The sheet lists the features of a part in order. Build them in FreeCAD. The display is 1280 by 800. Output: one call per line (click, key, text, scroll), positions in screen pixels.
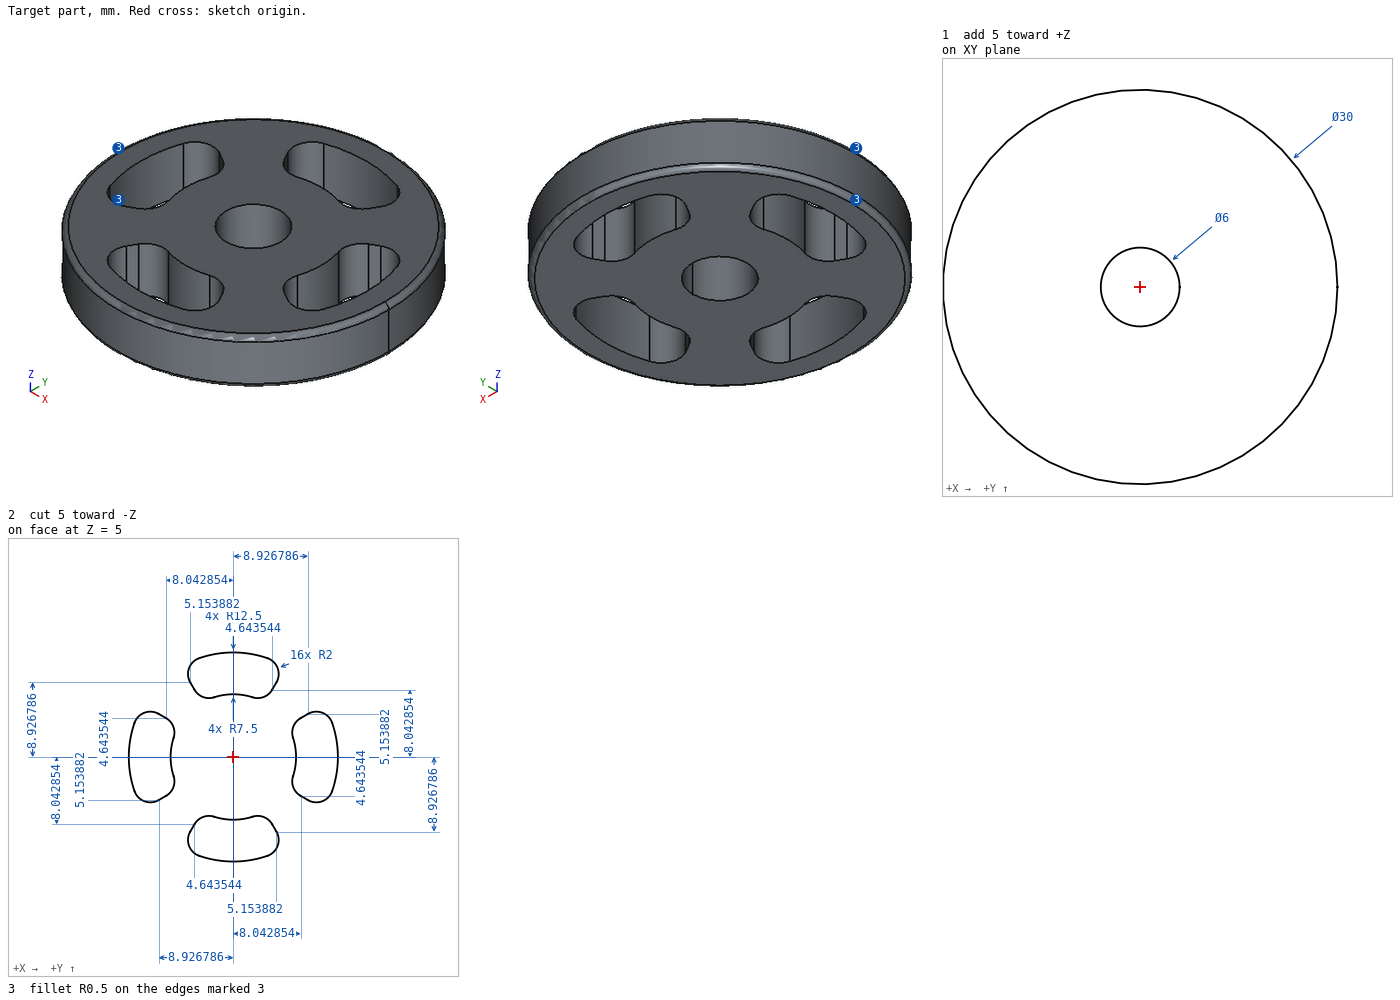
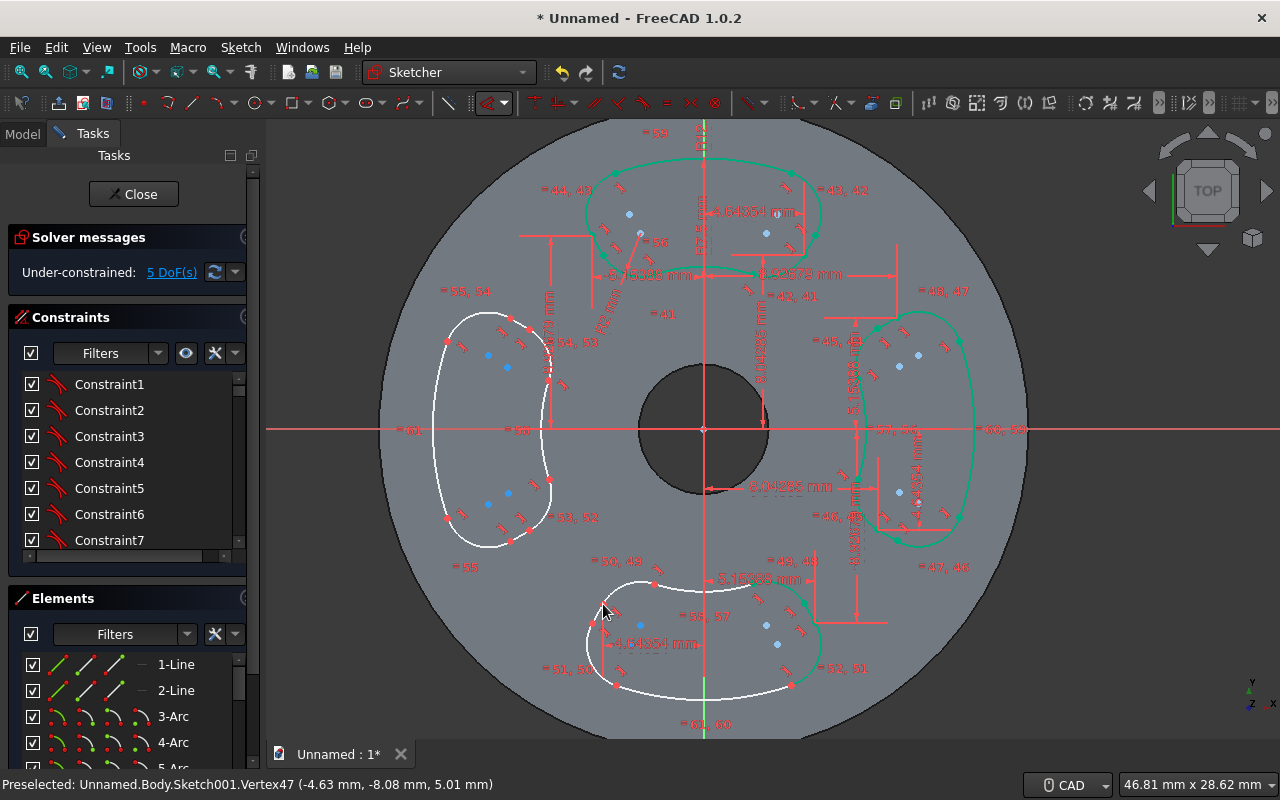
click(603, 604)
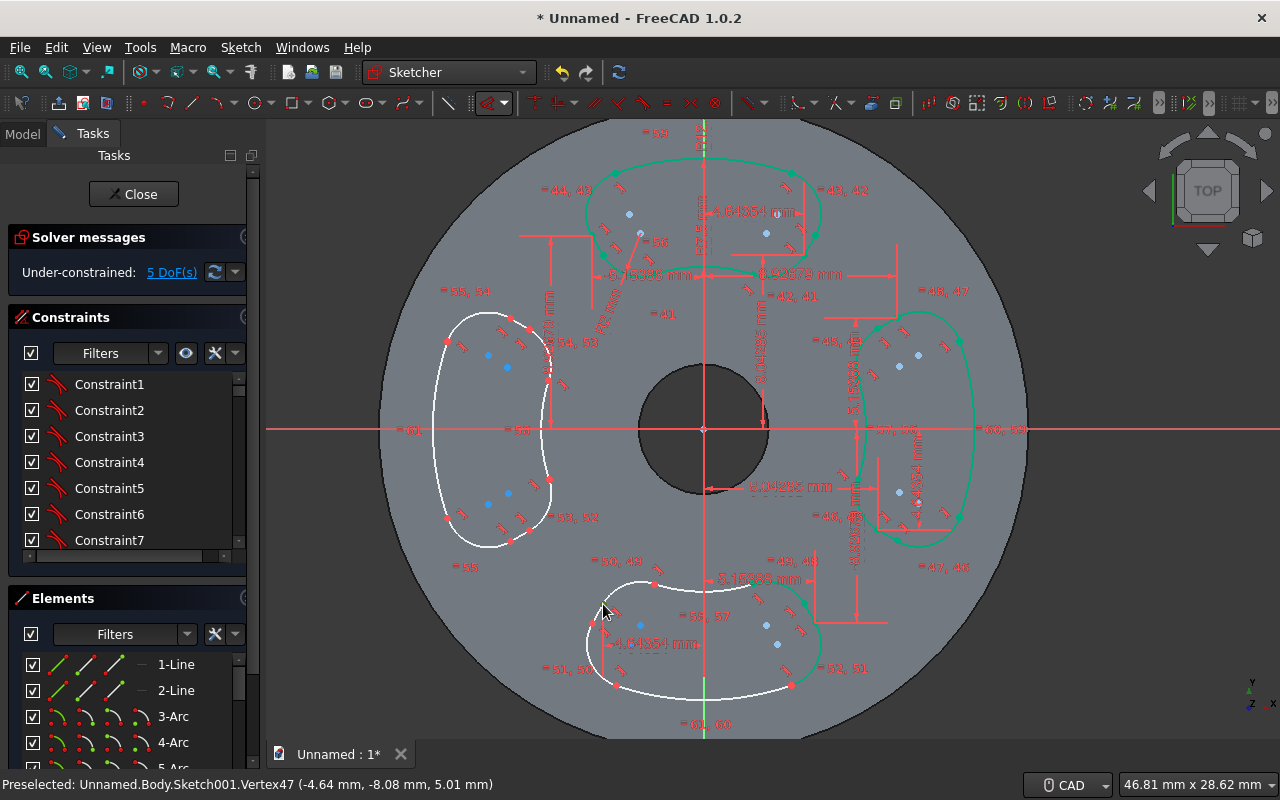
click(506, 104)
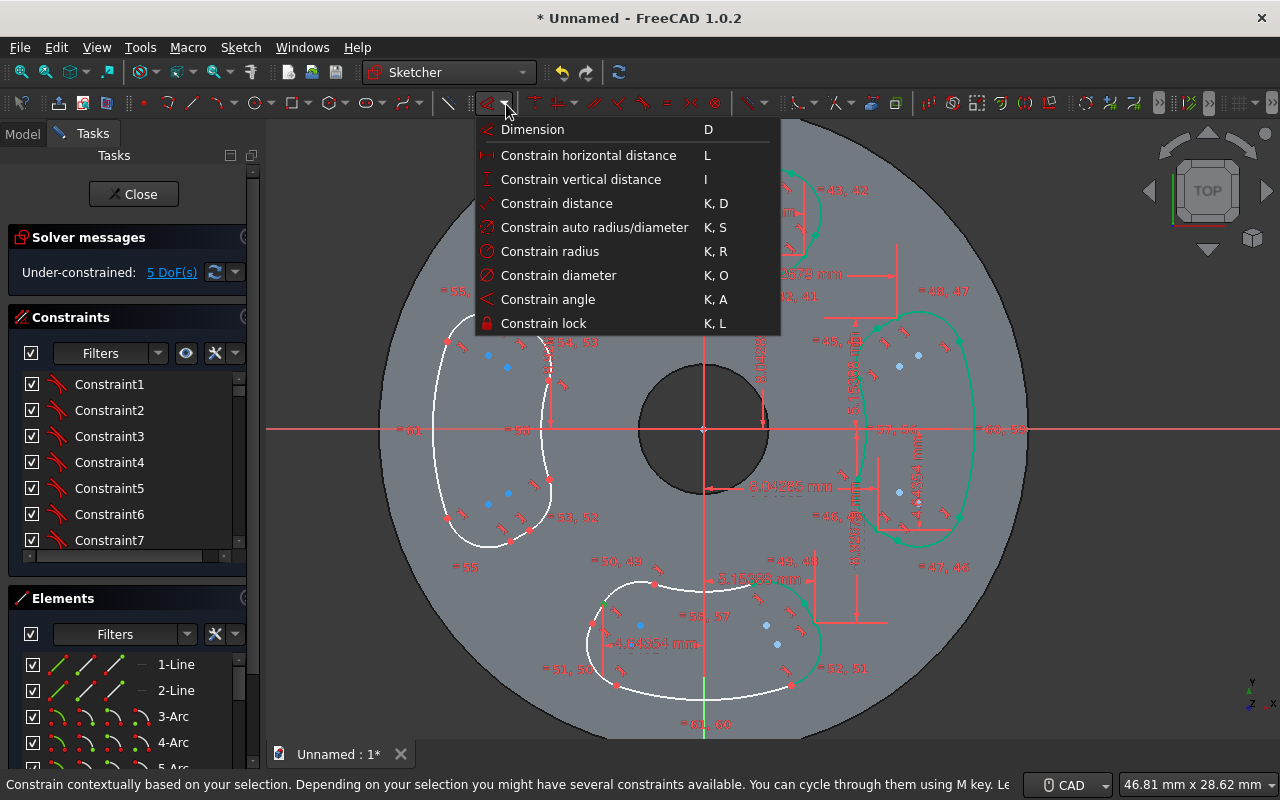
click(628, 179)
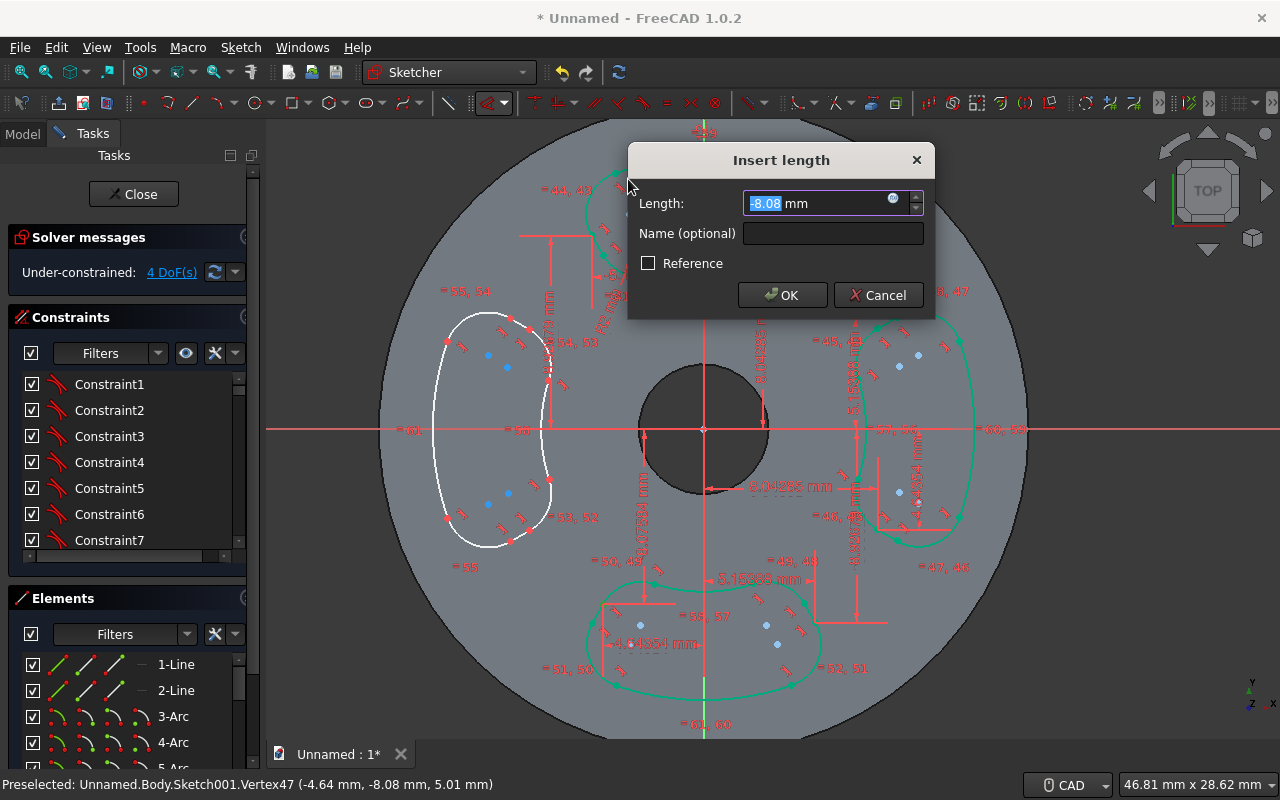
text(-8.042854)
key(Return)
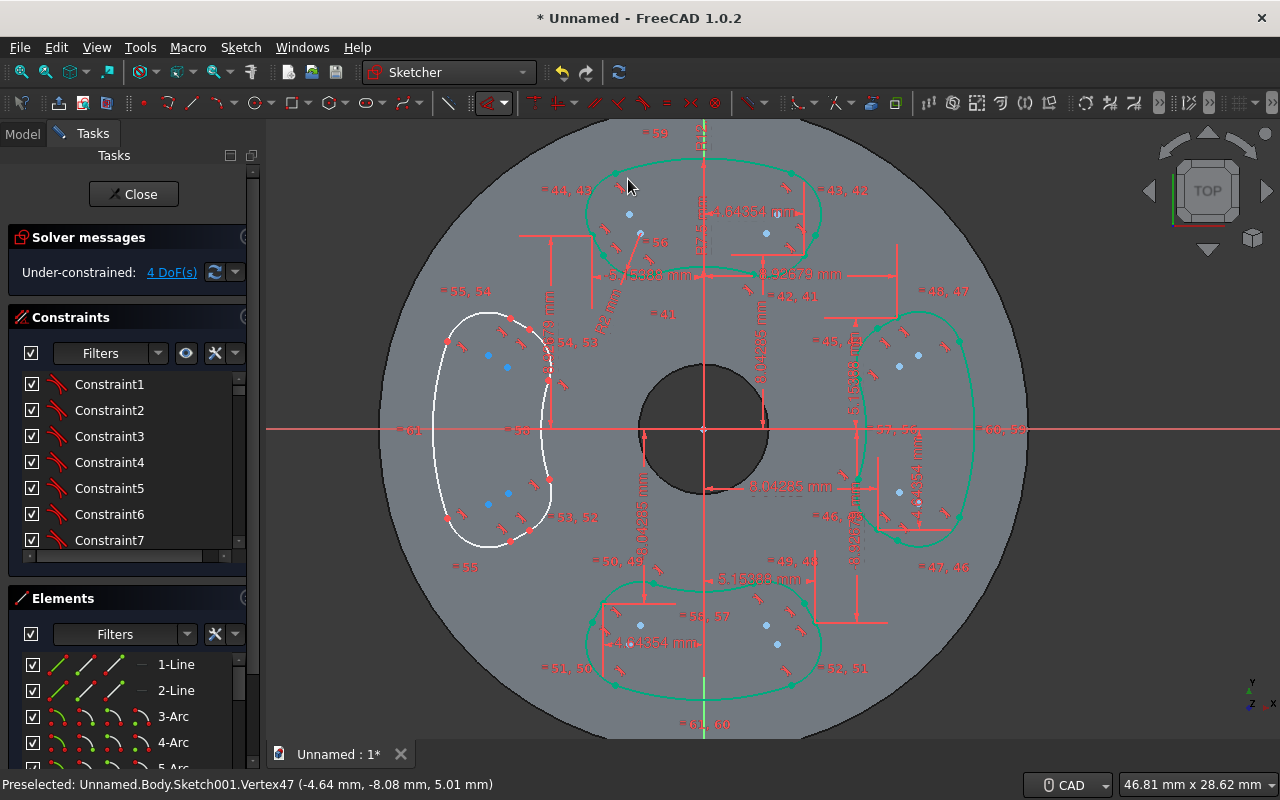
click(510, 542)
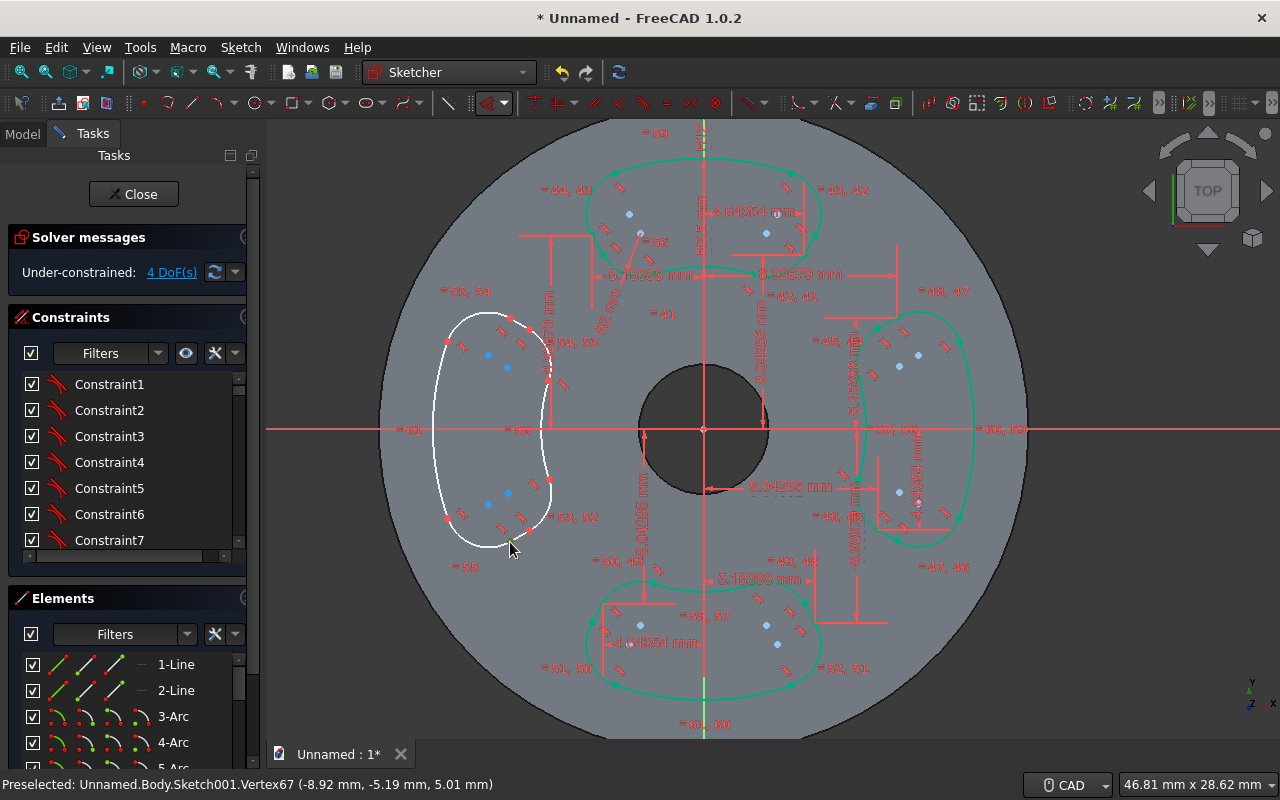
click(506, 104)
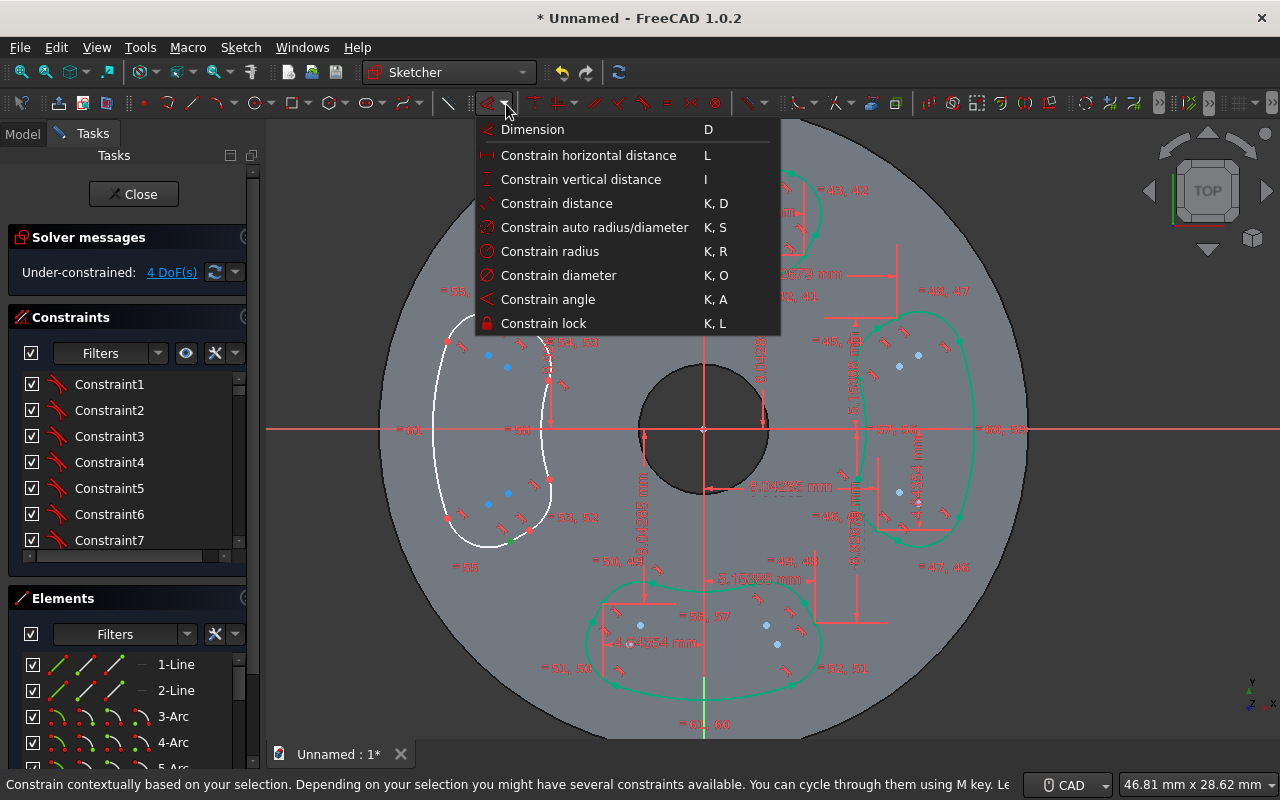
click(628, 155)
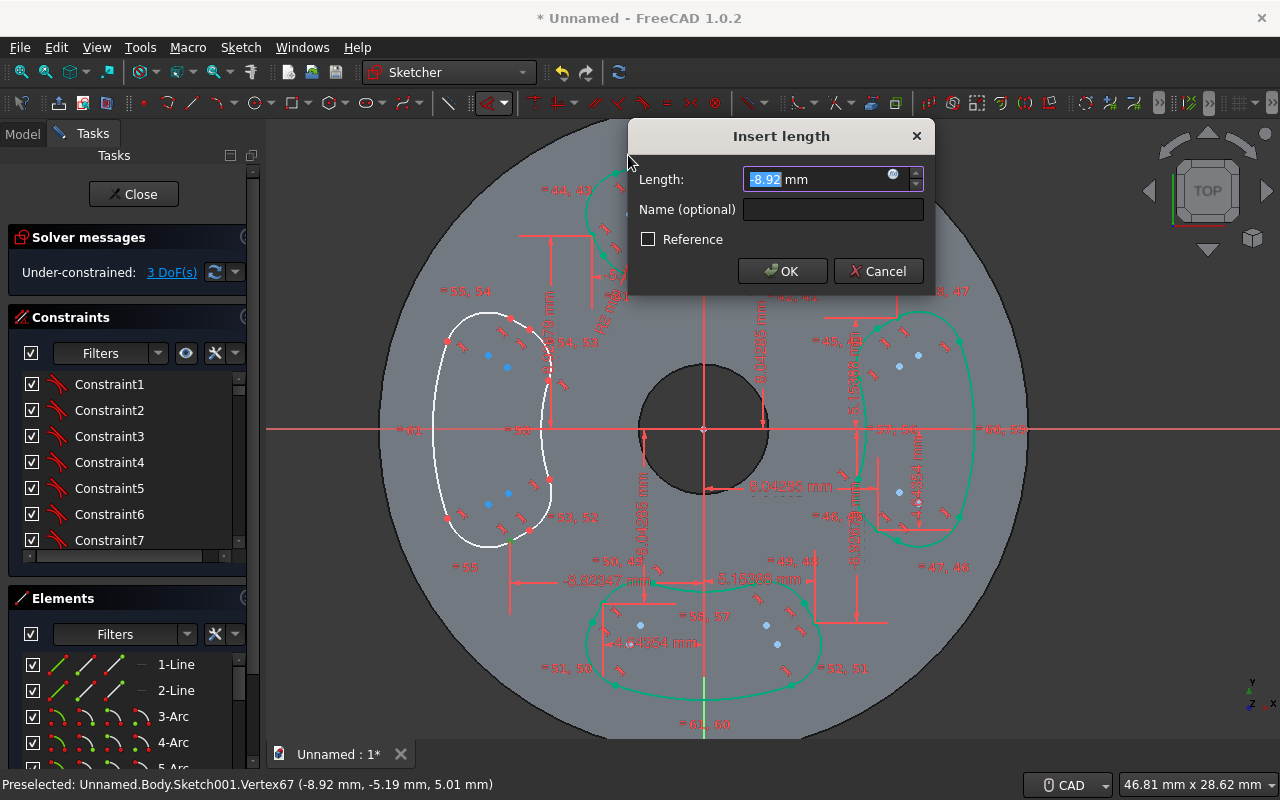
text(-8.926786)
key(Return)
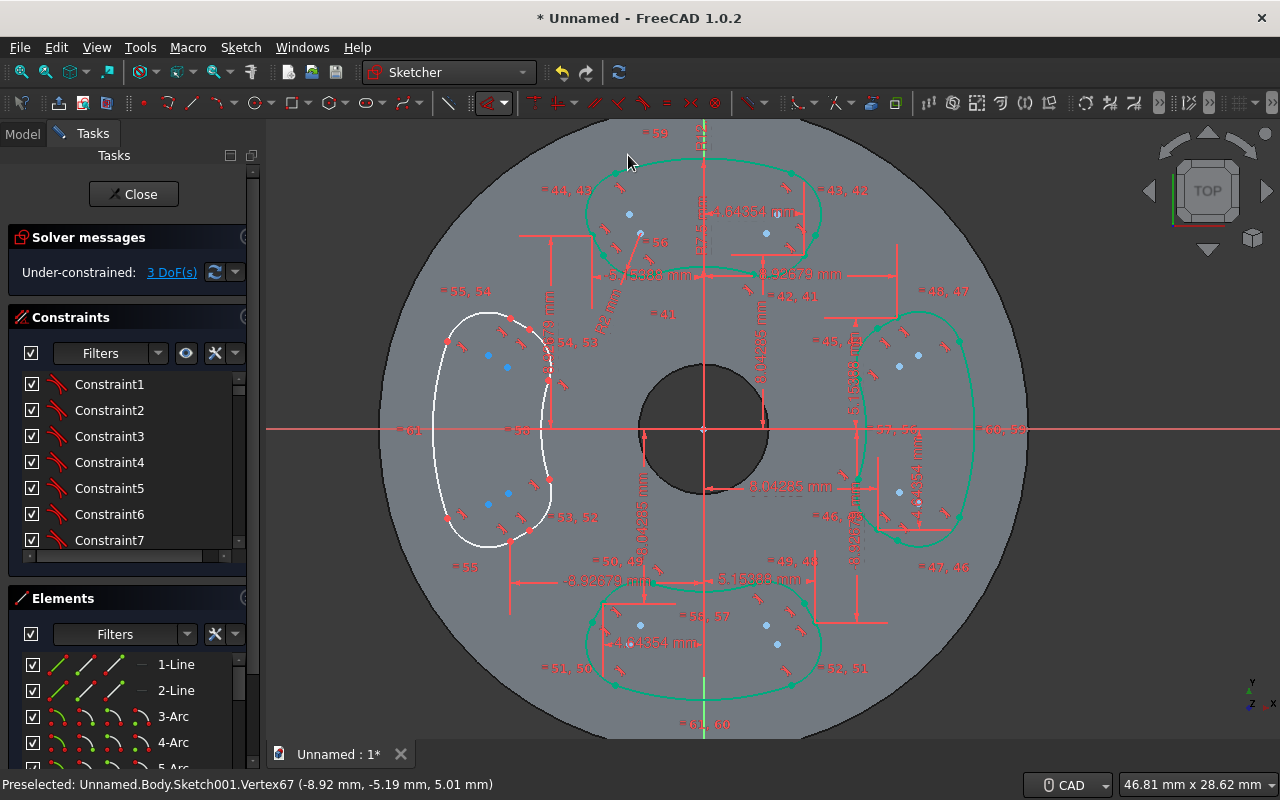
click(510, 542)